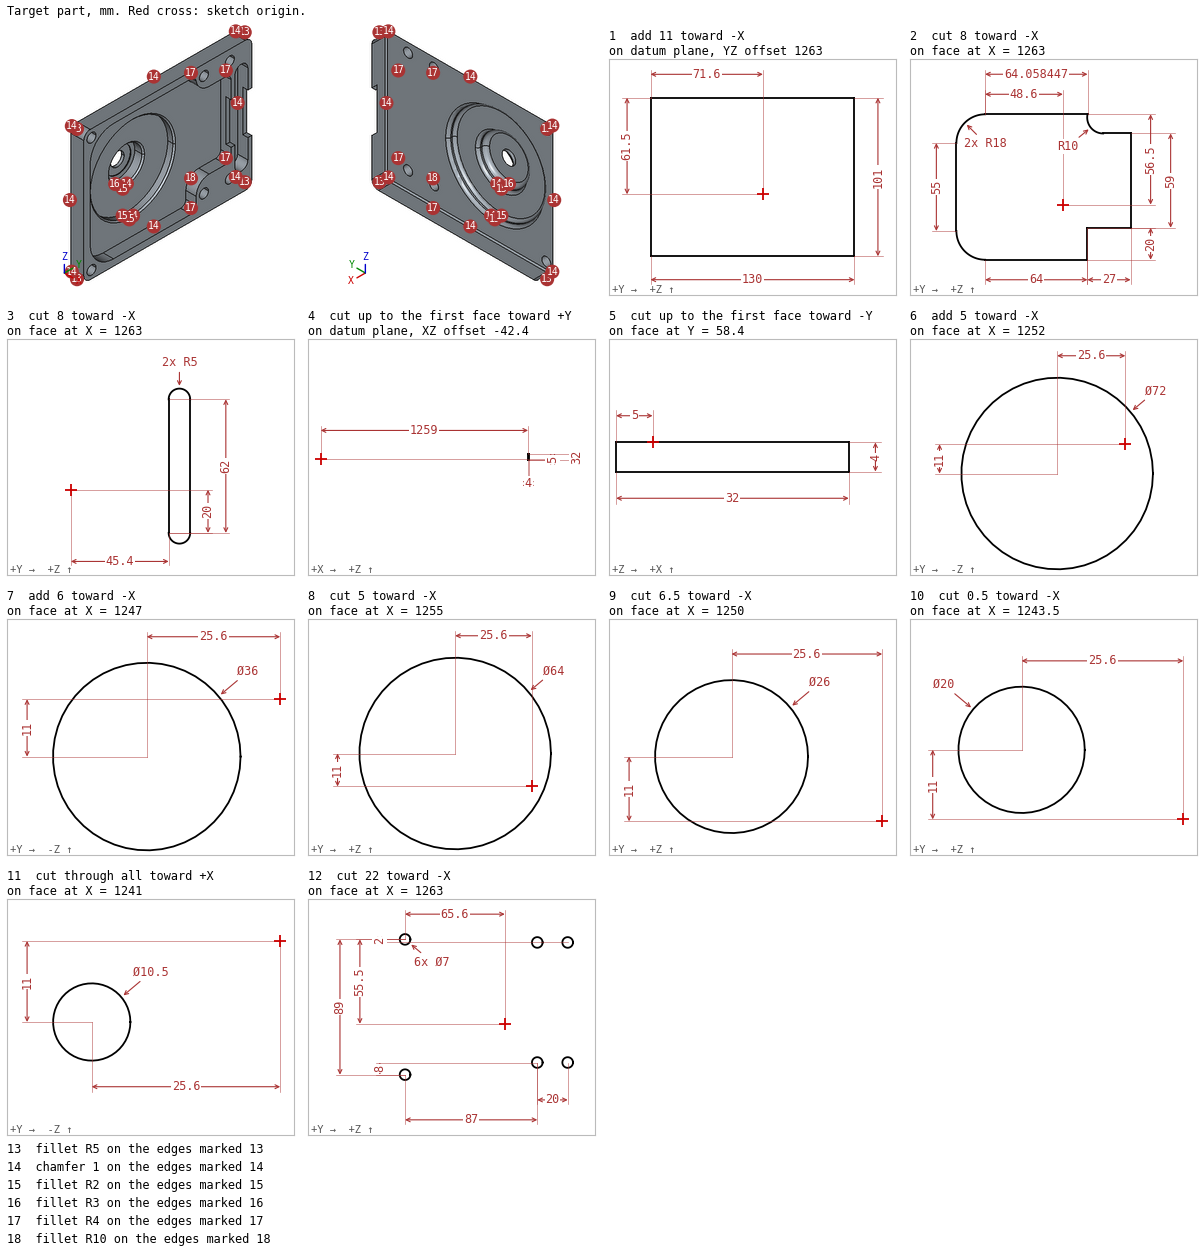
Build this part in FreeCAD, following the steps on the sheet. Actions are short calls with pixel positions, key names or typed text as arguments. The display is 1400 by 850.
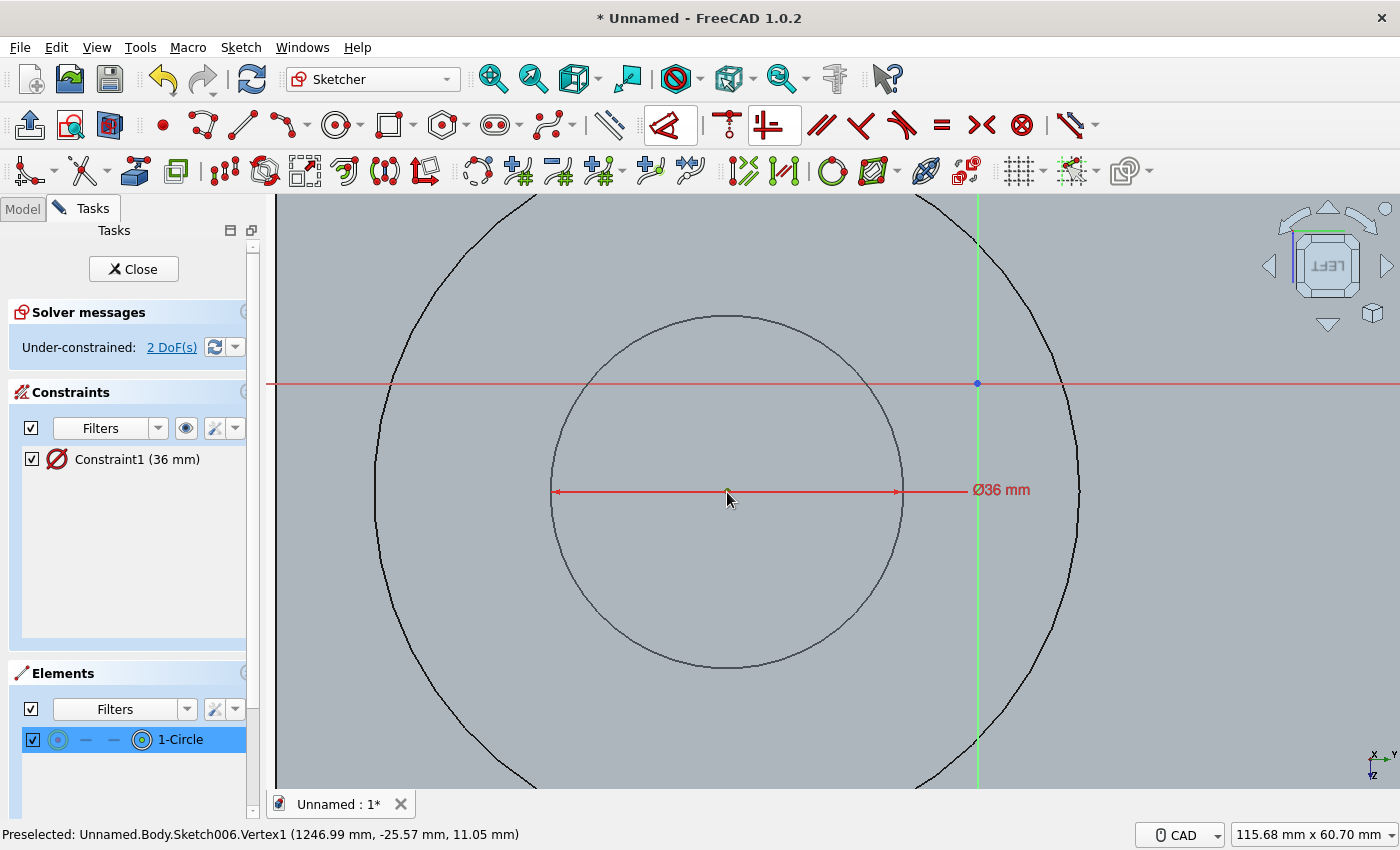
key(i)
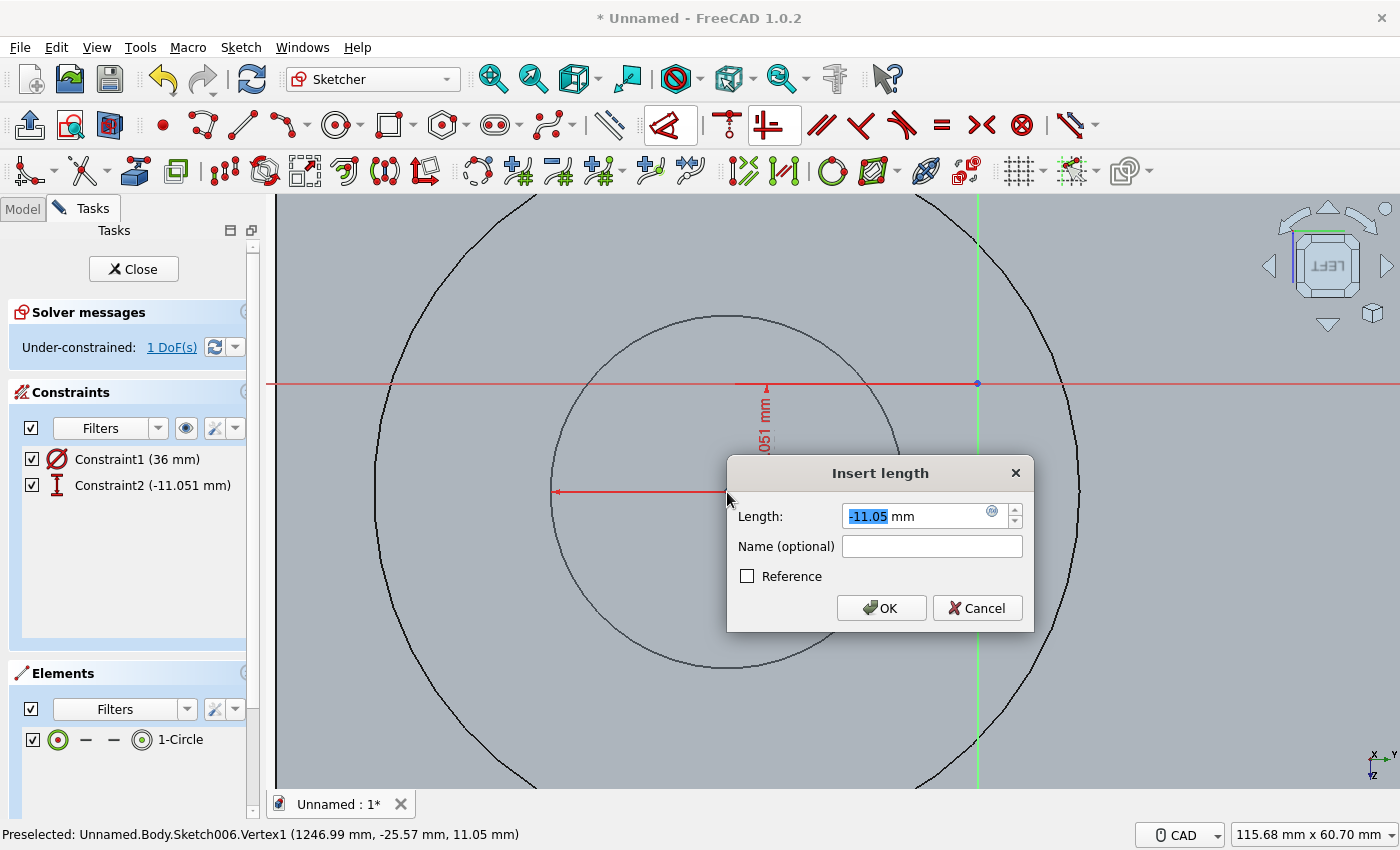
text(-11)
key(Return)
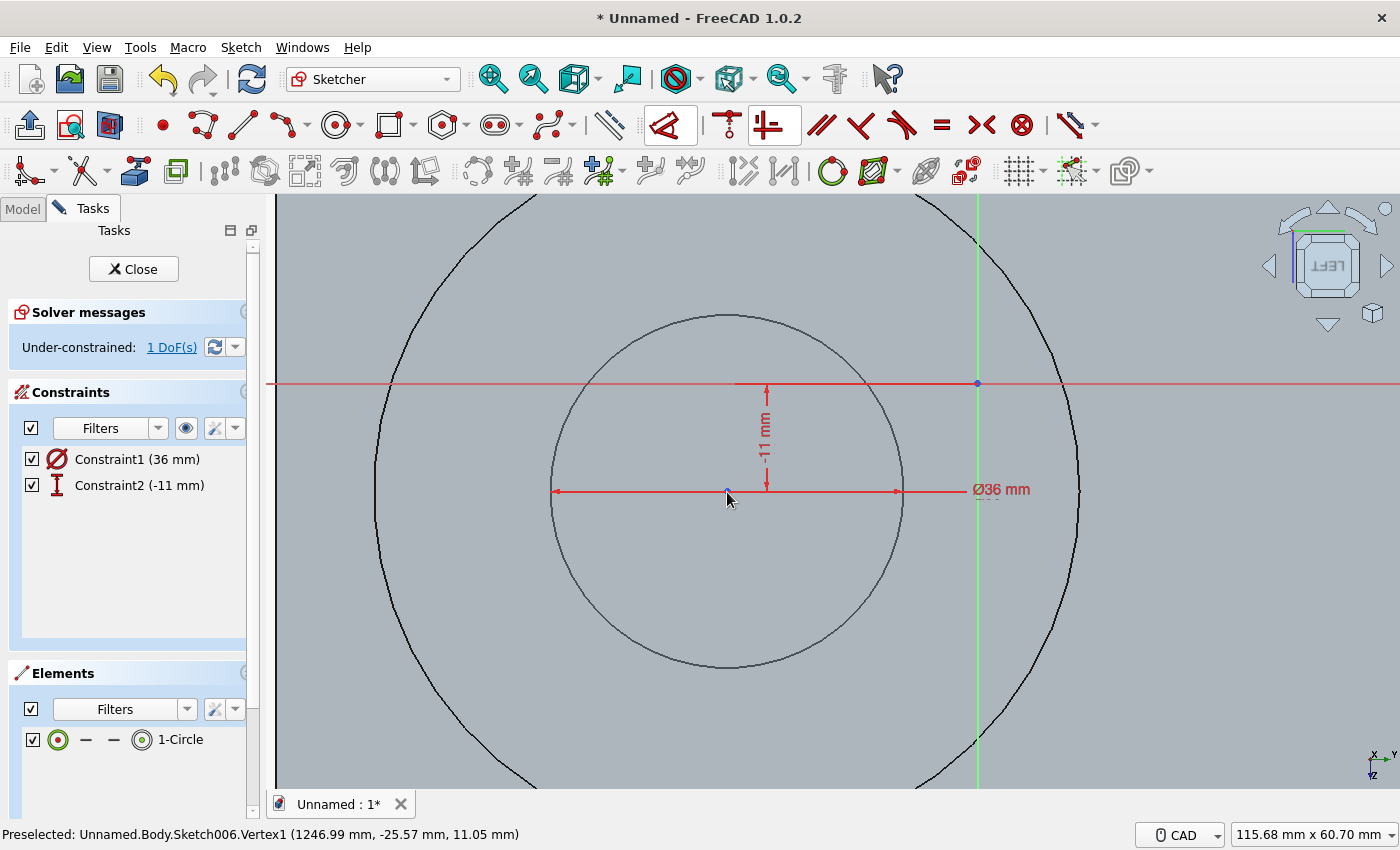
click(727, 491)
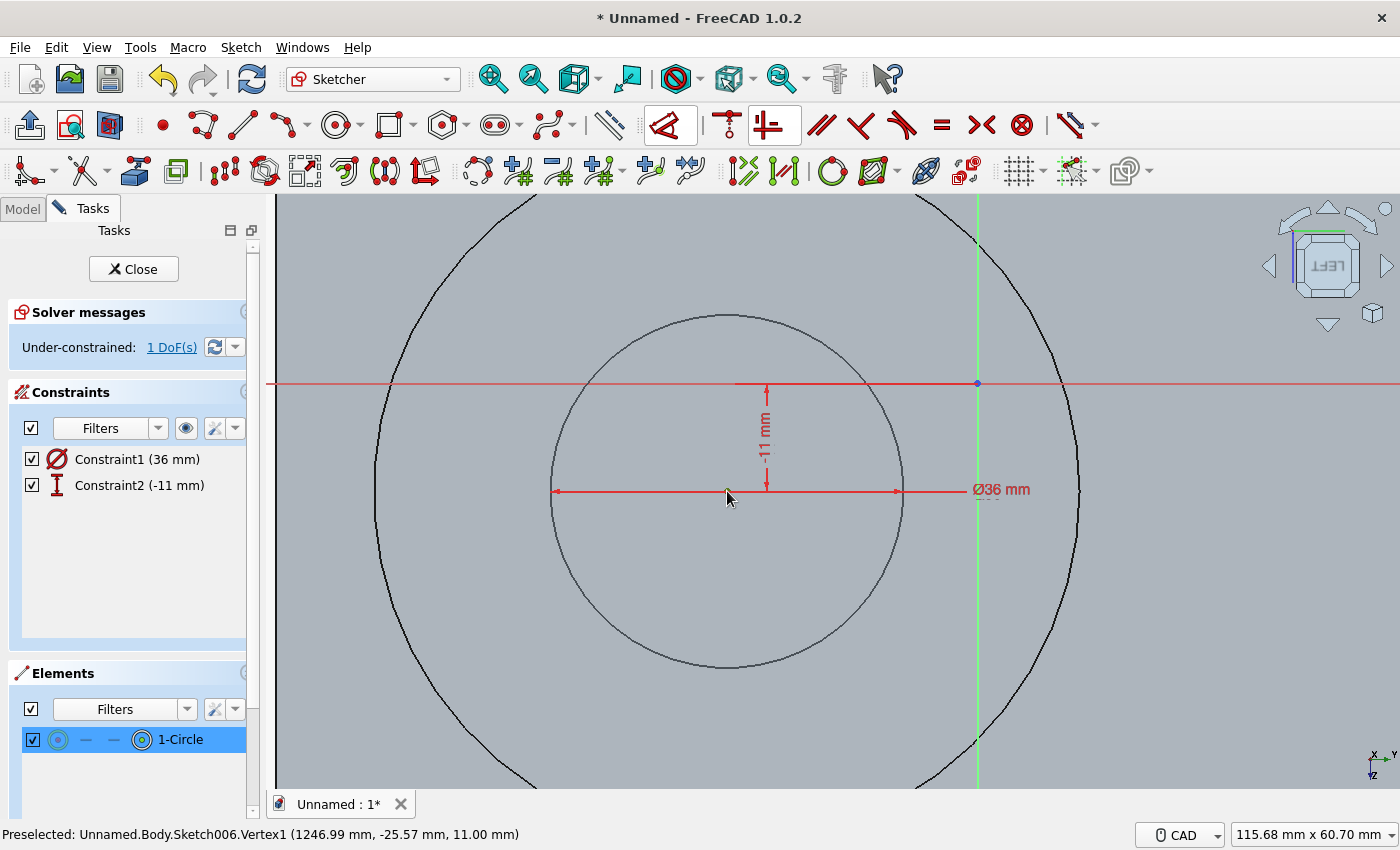
key(l)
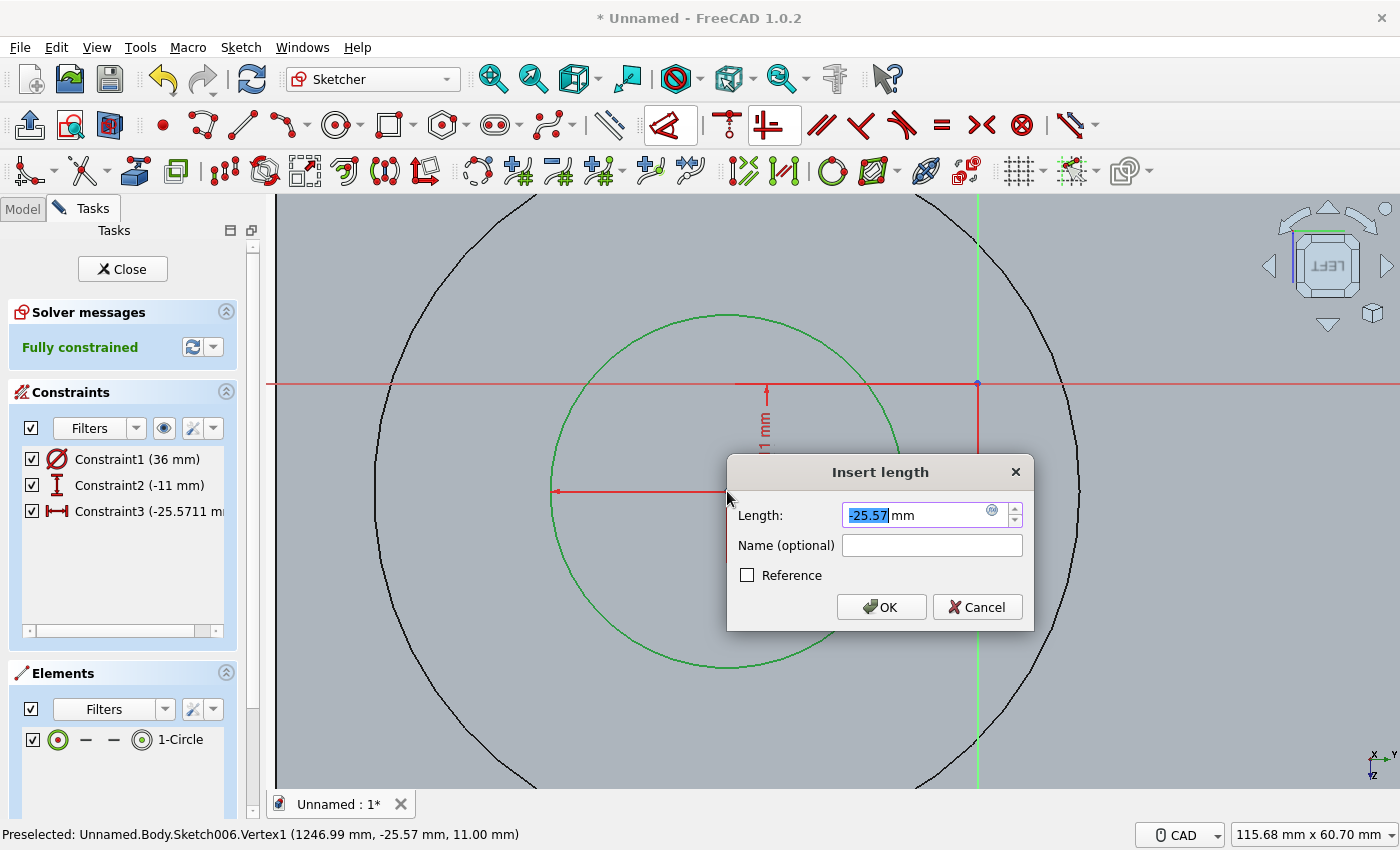
text(-25.6)
key(Return)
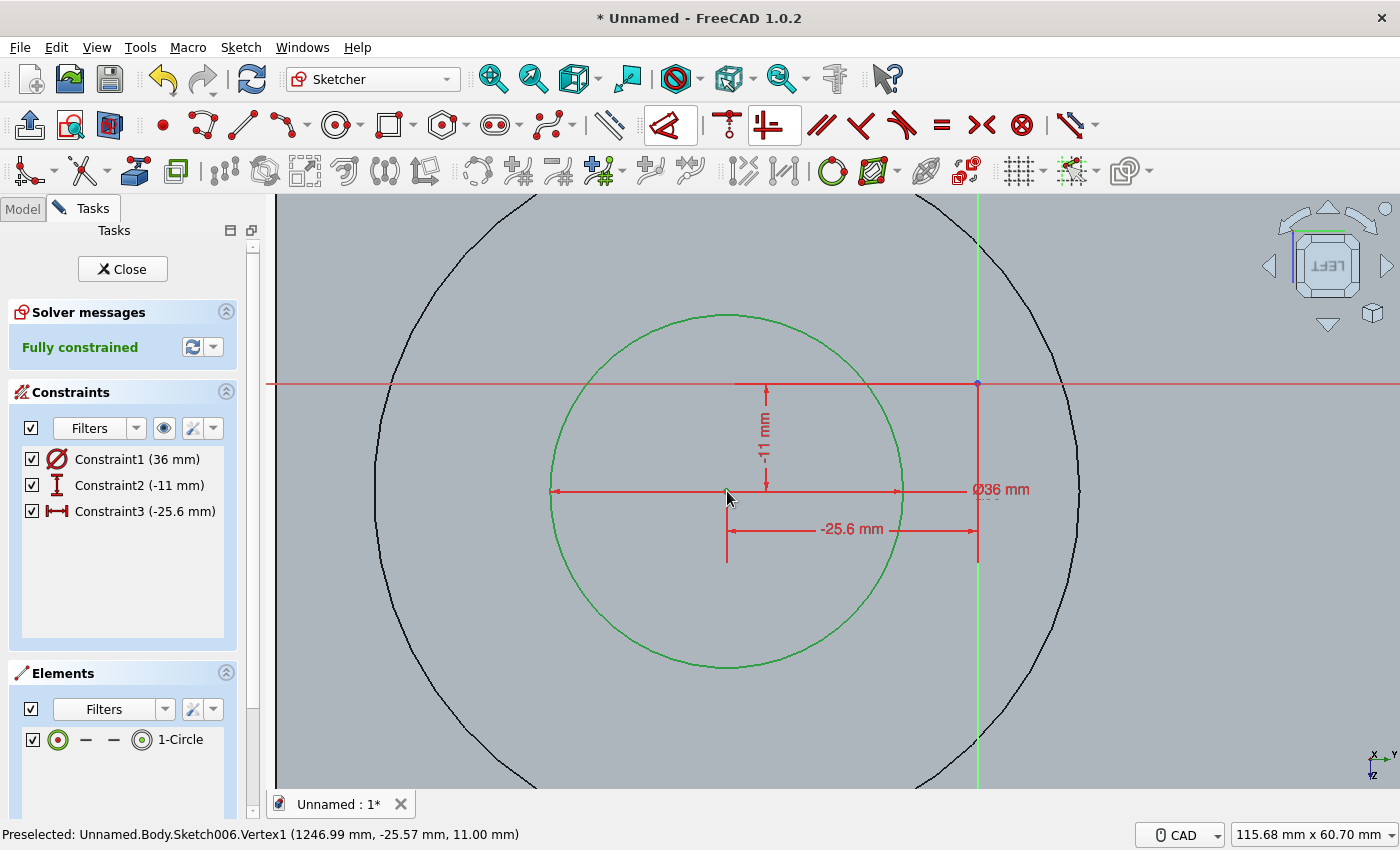
click(123, 269)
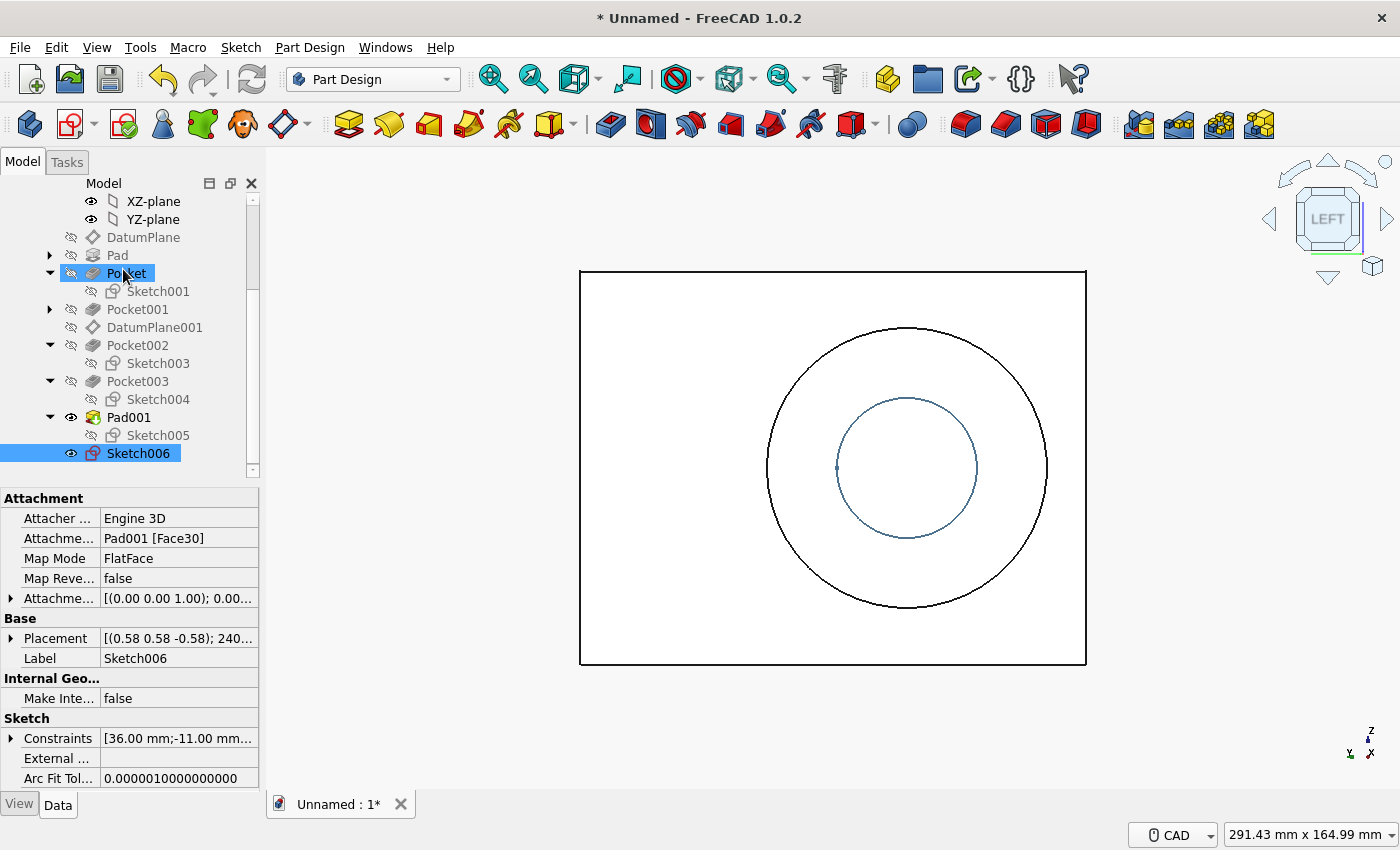
click(350, 124)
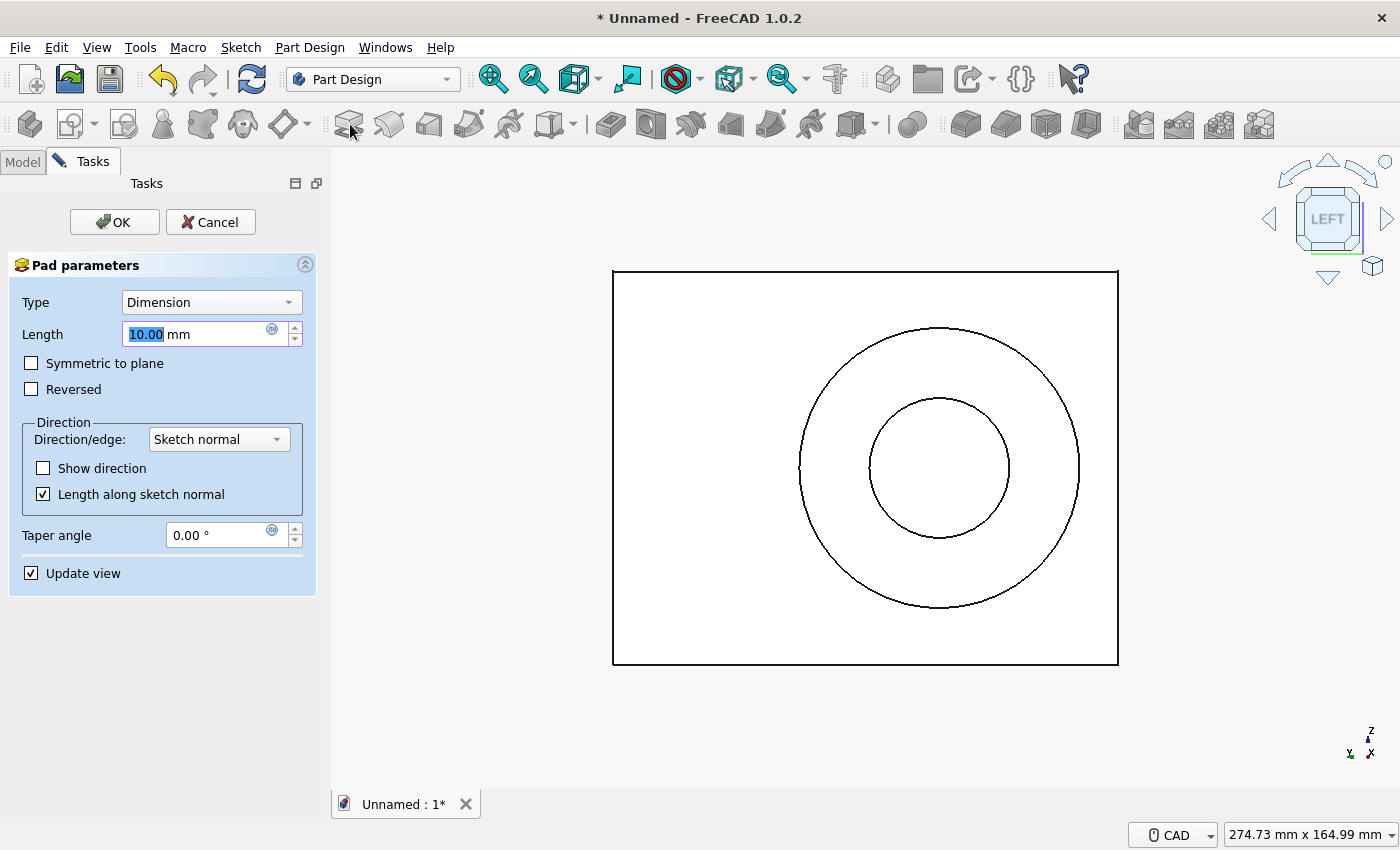
text(6)
key(Tab)